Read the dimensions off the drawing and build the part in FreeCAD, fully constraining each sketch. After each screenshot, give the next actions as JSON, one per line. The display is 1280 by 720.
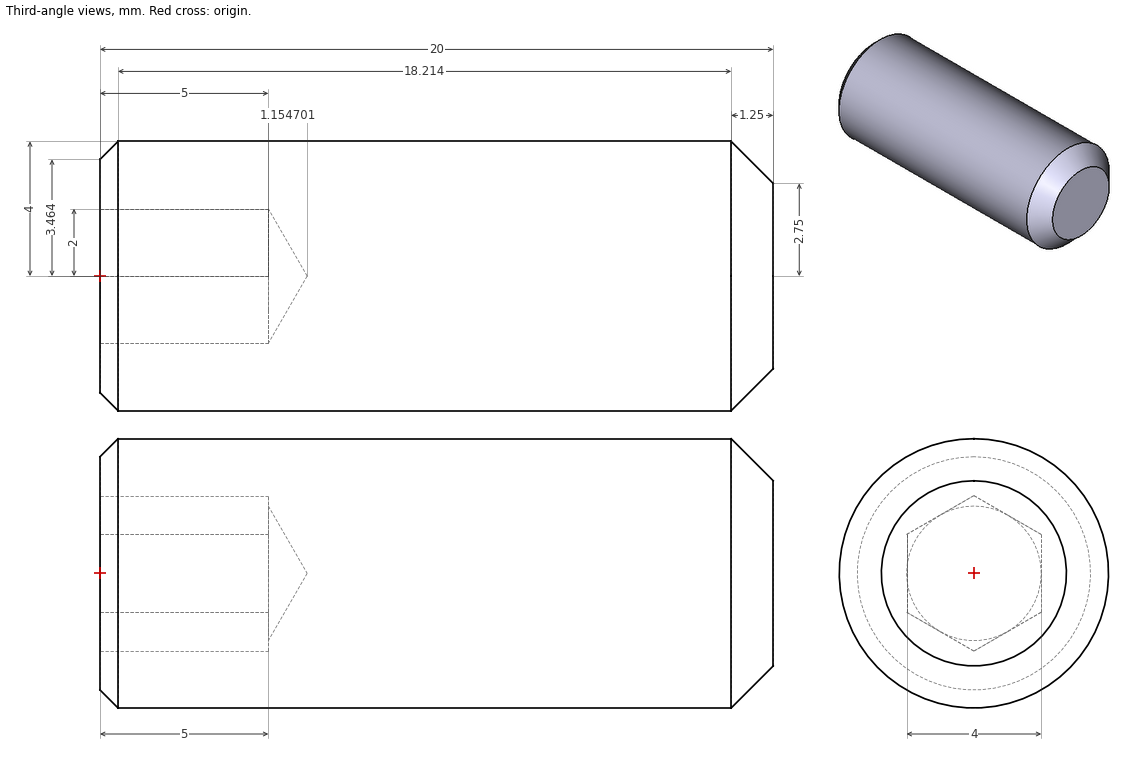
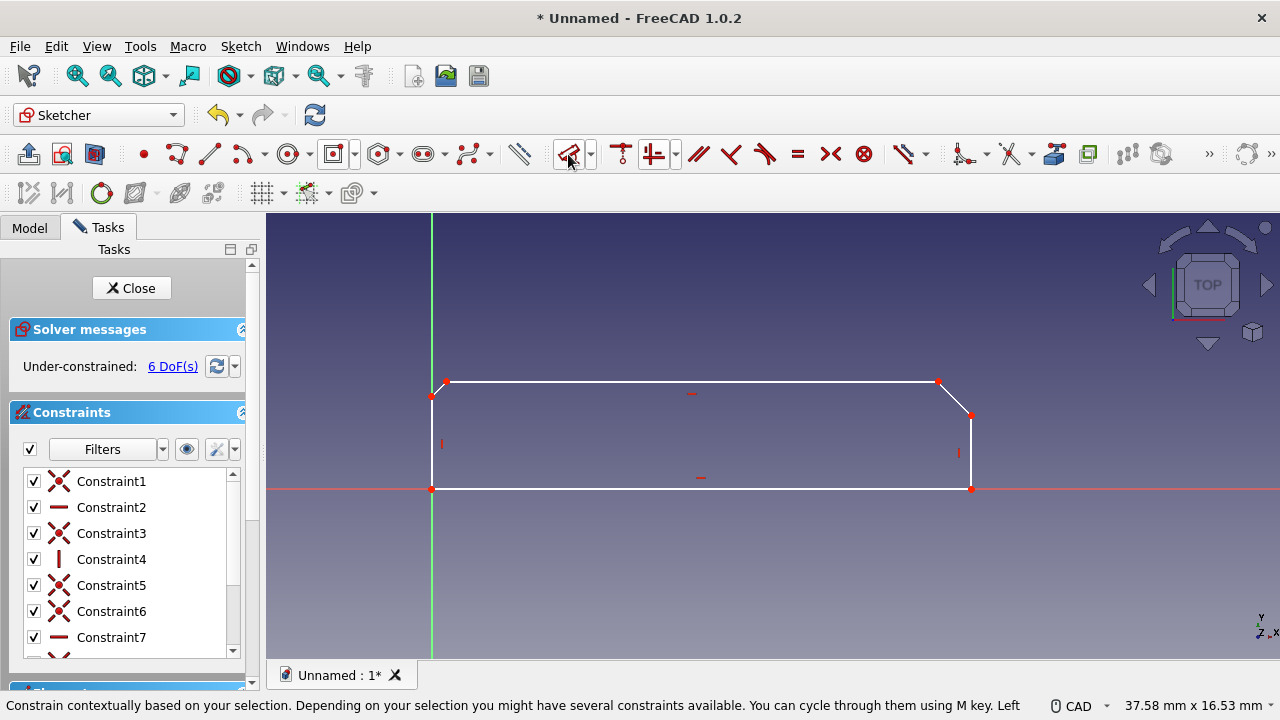
{"action": "left_click", "coordinate": [594, 489]}
{"action": "left_click", "coordinate": [701, 523]}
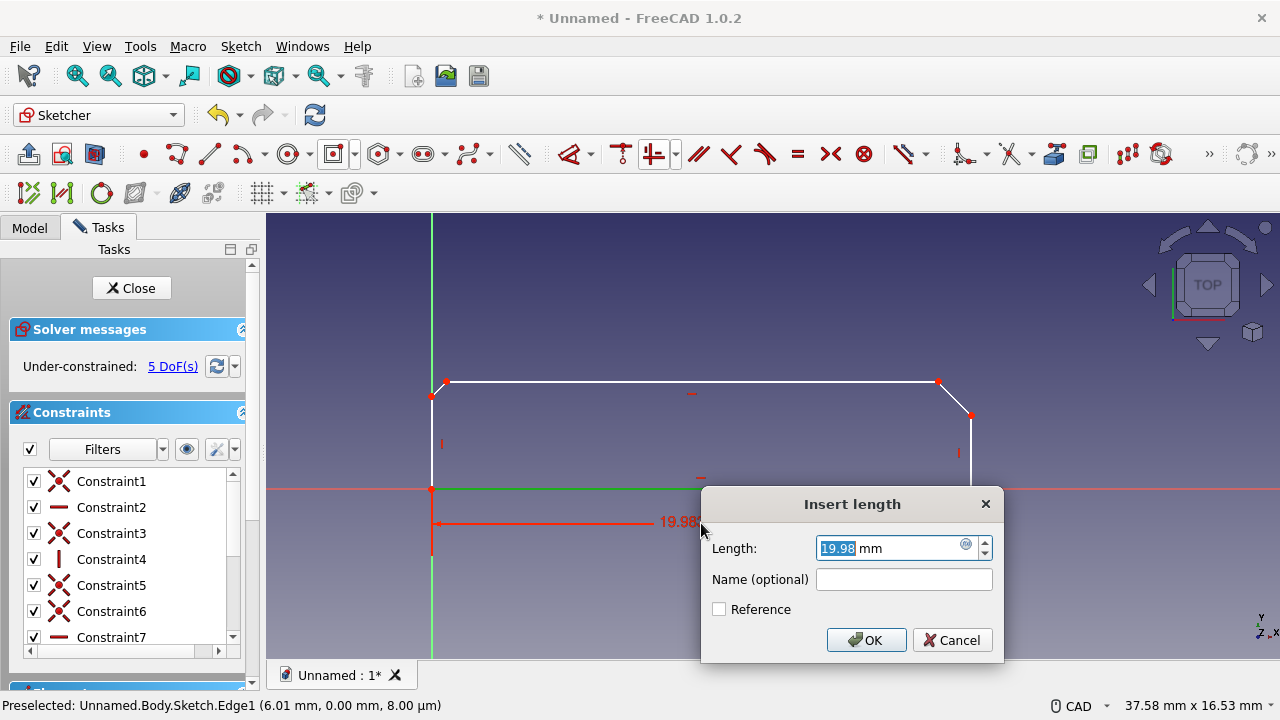
{"action": "type", "text": "20"}
{"action": "key", "text": "Return"}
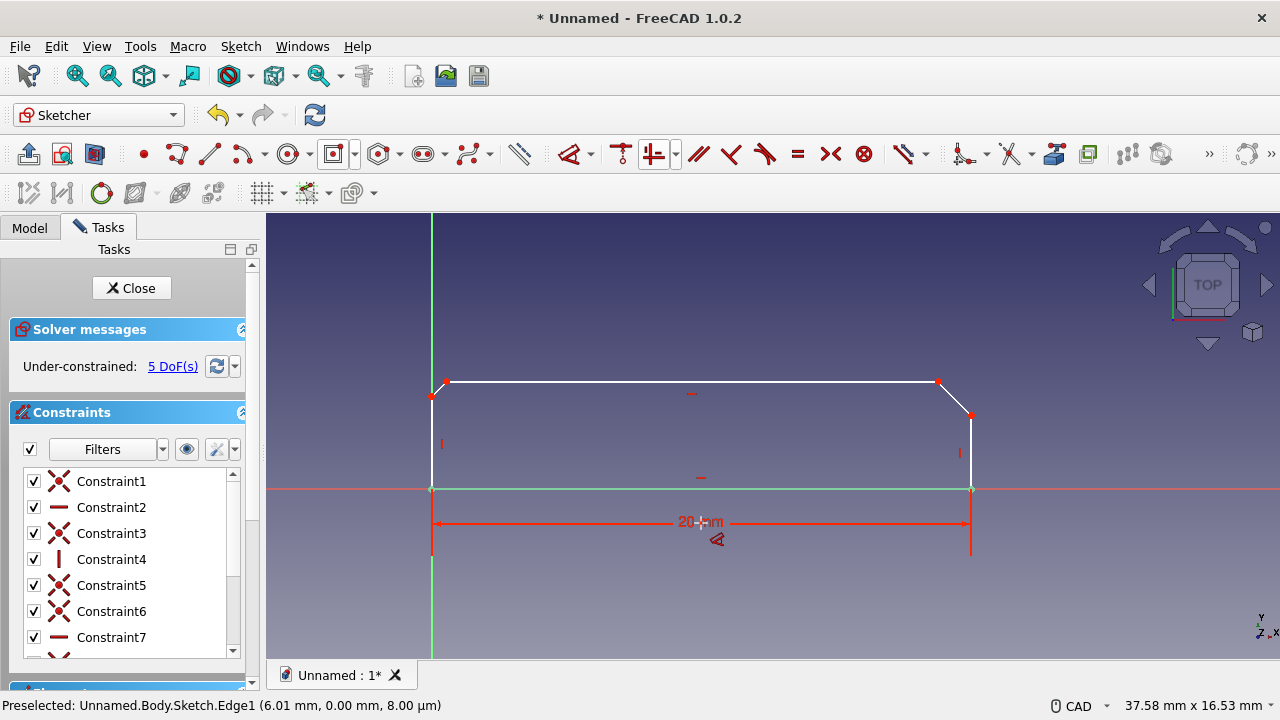
{"action": "left_click", "coordinate": [938, 382]}
{"action": "left_click", "coordinate": [398, 436]}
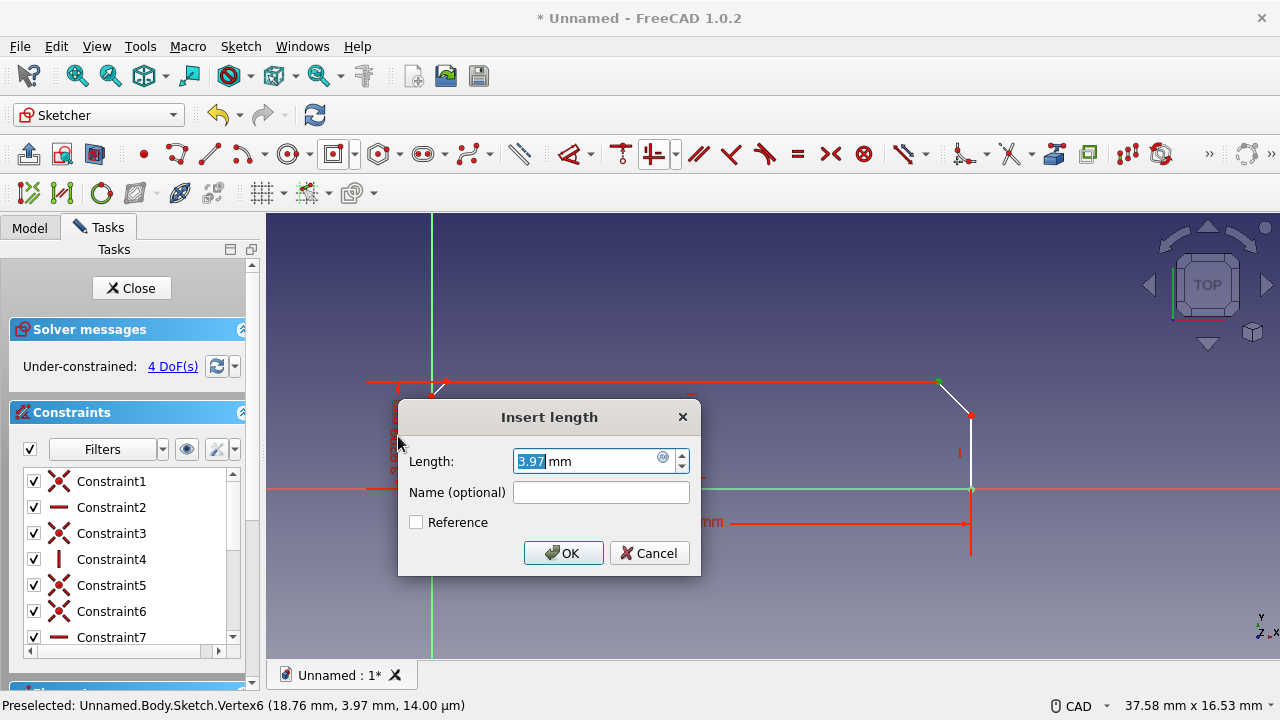
{"action": "type", "text": "4"}
{"action": "key", "text": "Return"}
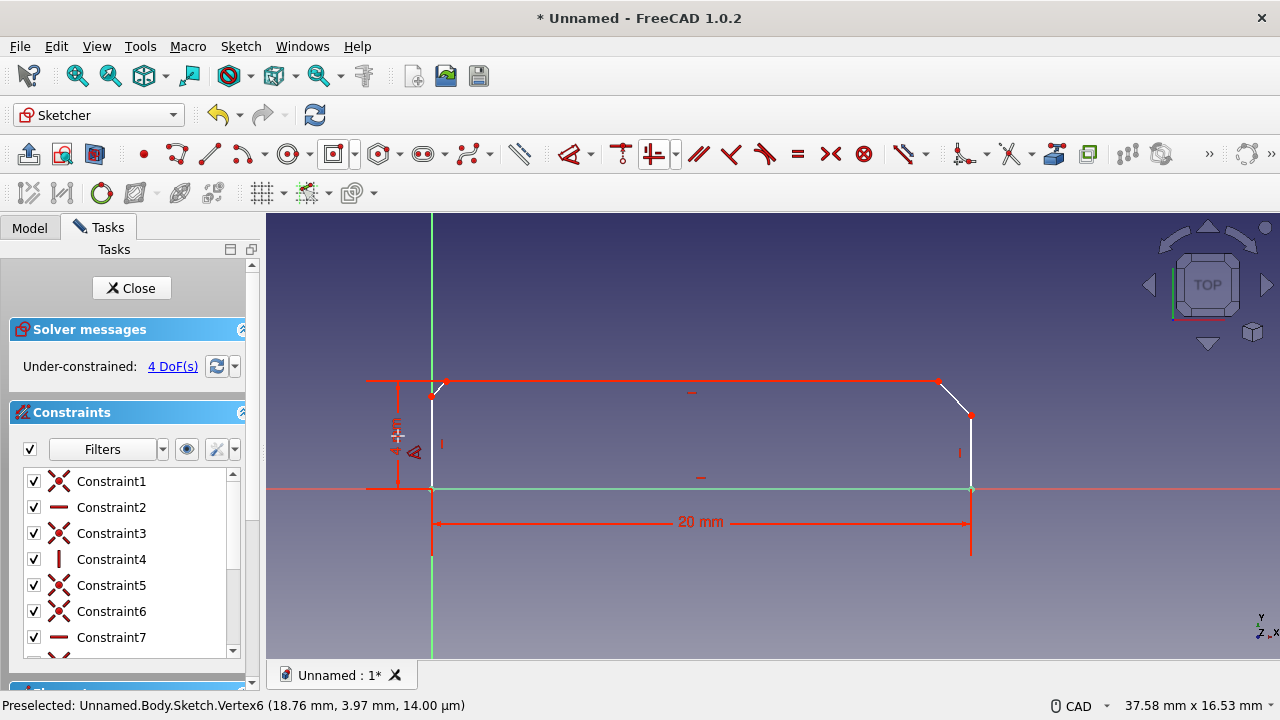
{"action": "left_click", "coordinate": [971, 467]}
{"action": "left_click", "coordinate": [1005, 453]}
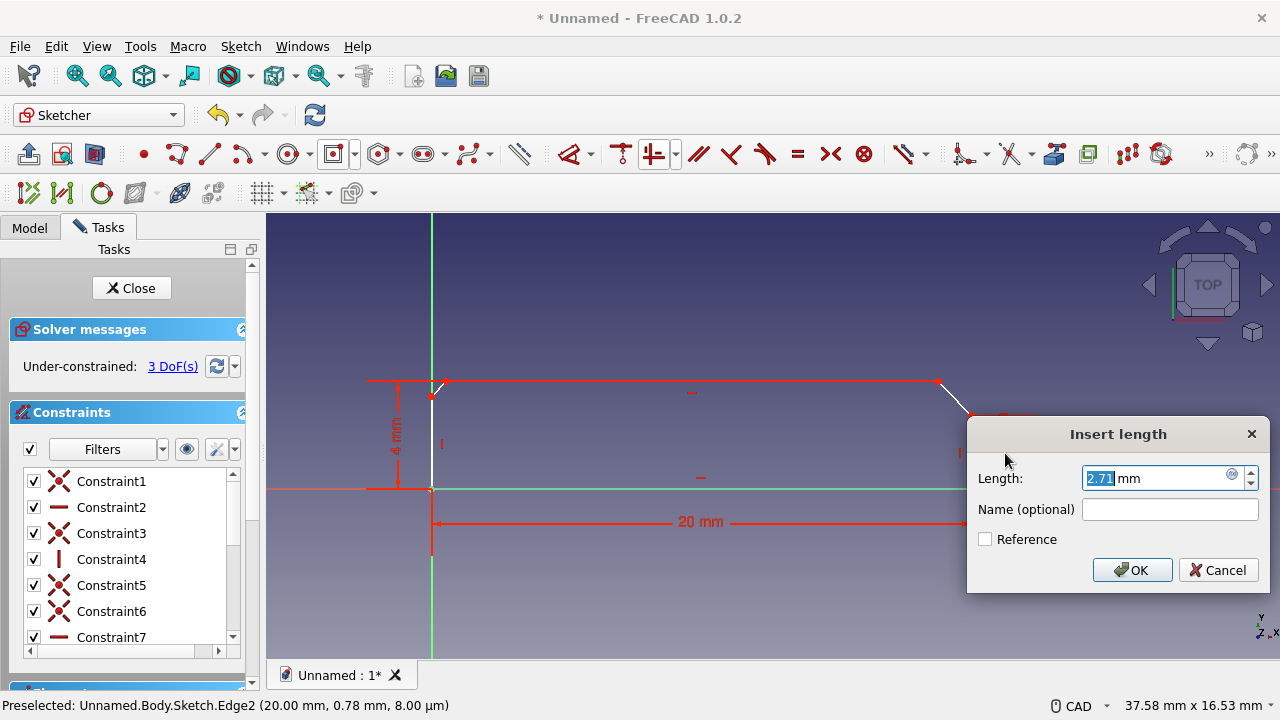
{"action": "type", "text": "2.75"}
{"action": "key", "text": "Return"}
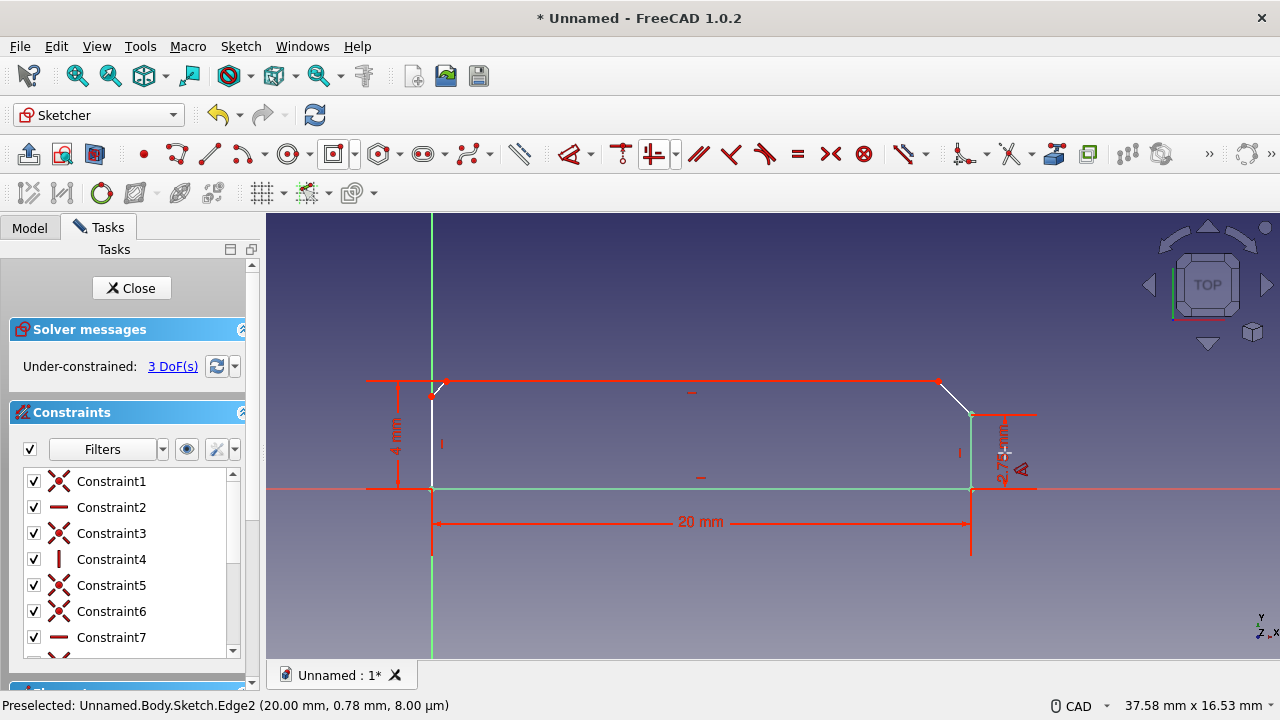
{"action": "left_click", "coordinate": [432, 425]}
{"action": "left_click", "coordinate": [398, 464]}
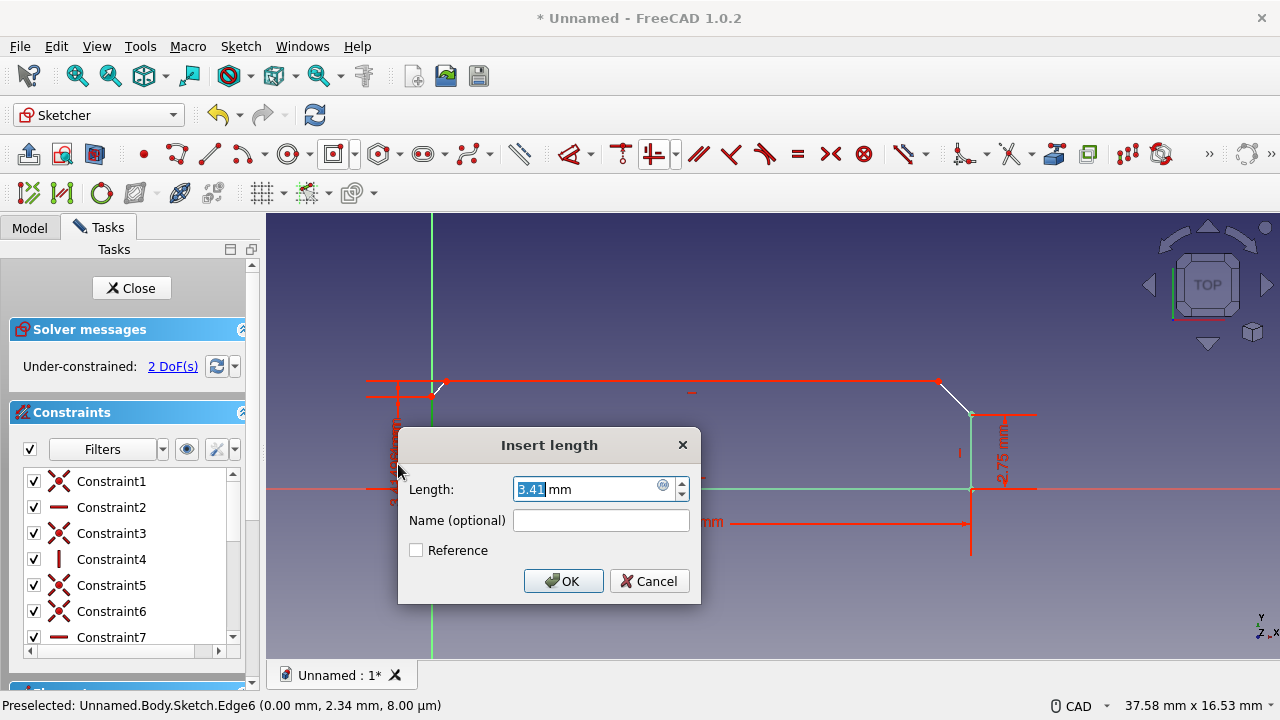
{"action": "type", "text": "3.464"}
{"action": "key", "text": "Return"}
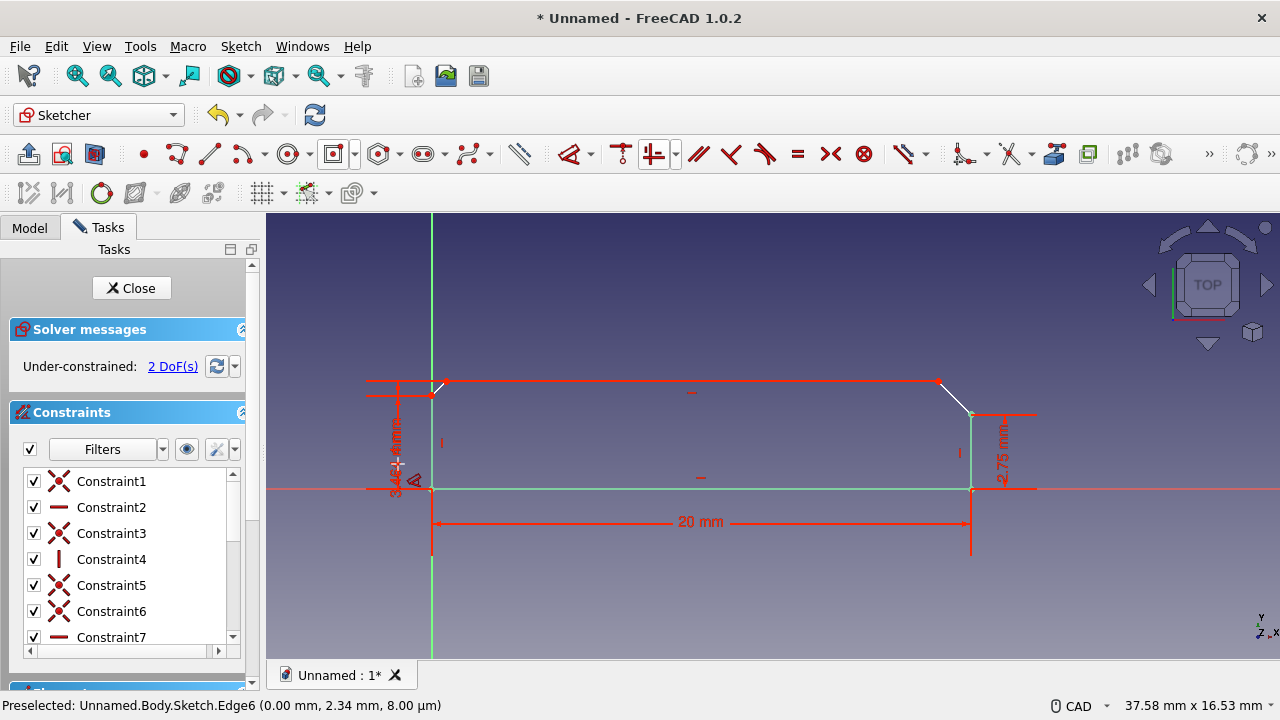
{"action": "left_click", "coordinate": [961, 405]}
{"action": "left_click", "coordinate": [955, 347]}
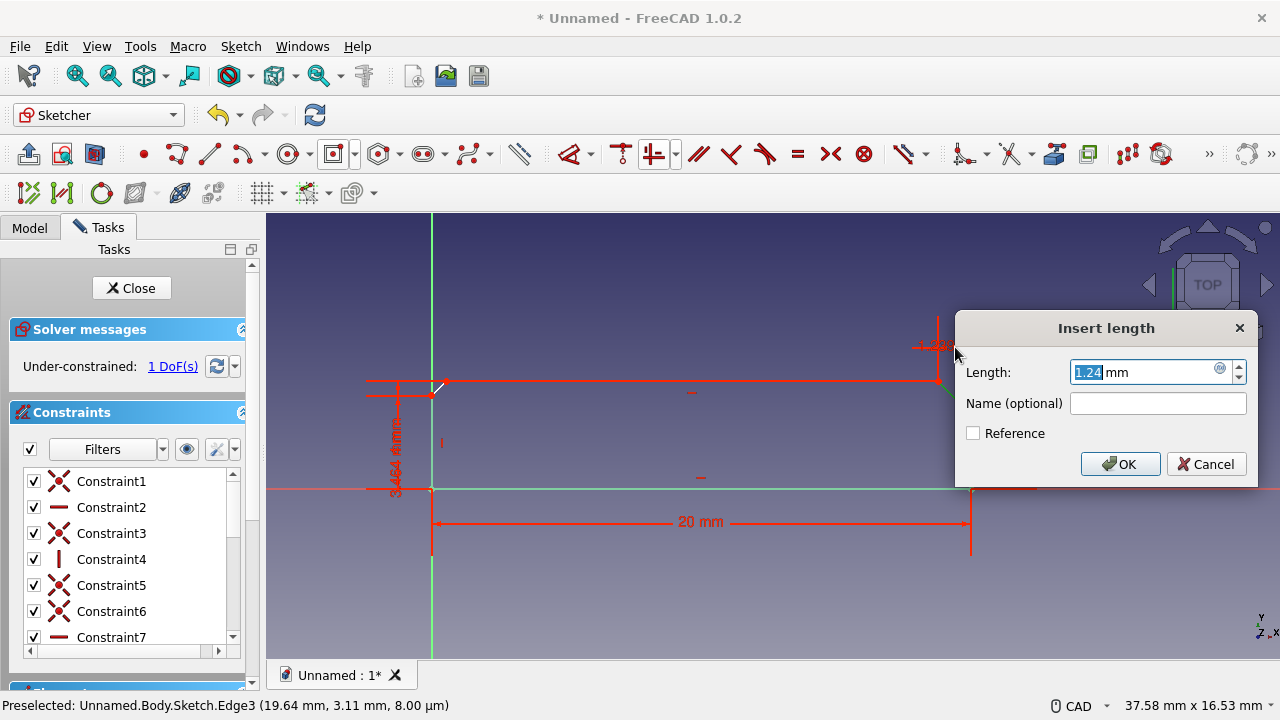
{"action": "type", "text": "1.25"}
{"action": "key", "text": "Return"}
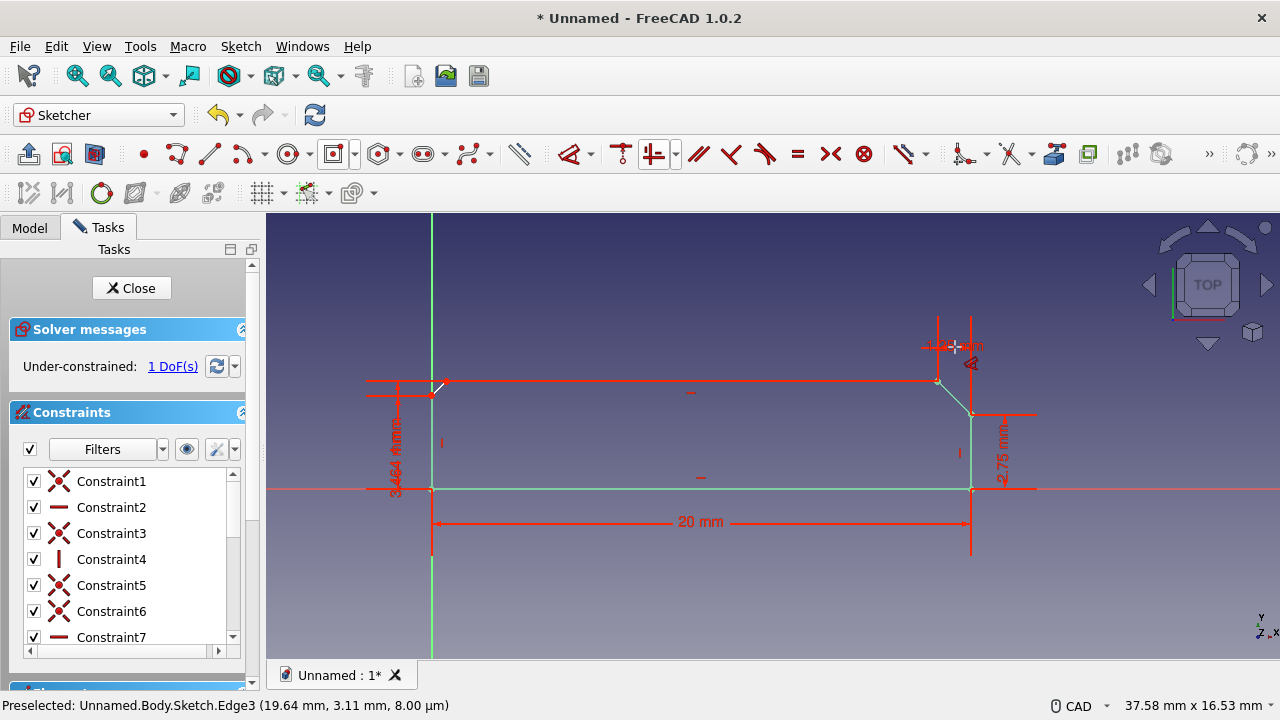
{"action": "left_click", "coordinate": [790, 381]}
{"action": "left_click", "coordinate": [692, 347]}